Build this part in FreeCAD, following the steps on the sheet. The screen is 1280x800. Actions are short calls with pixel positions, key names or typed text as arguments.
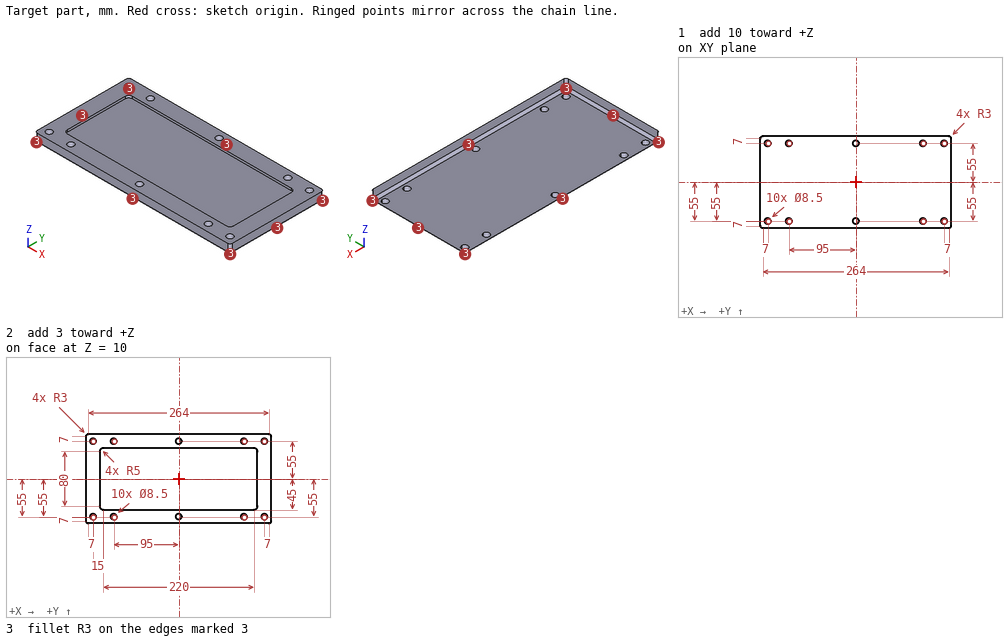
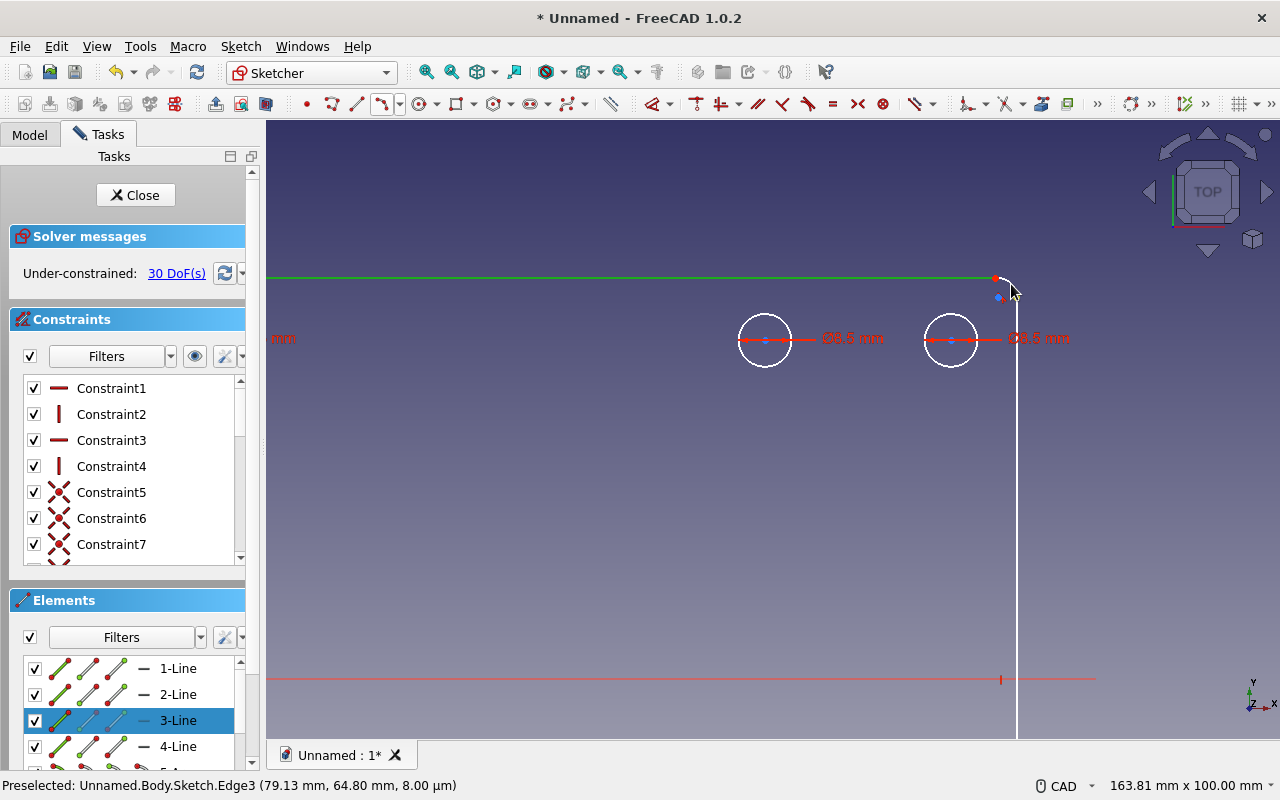
click(1010, 283)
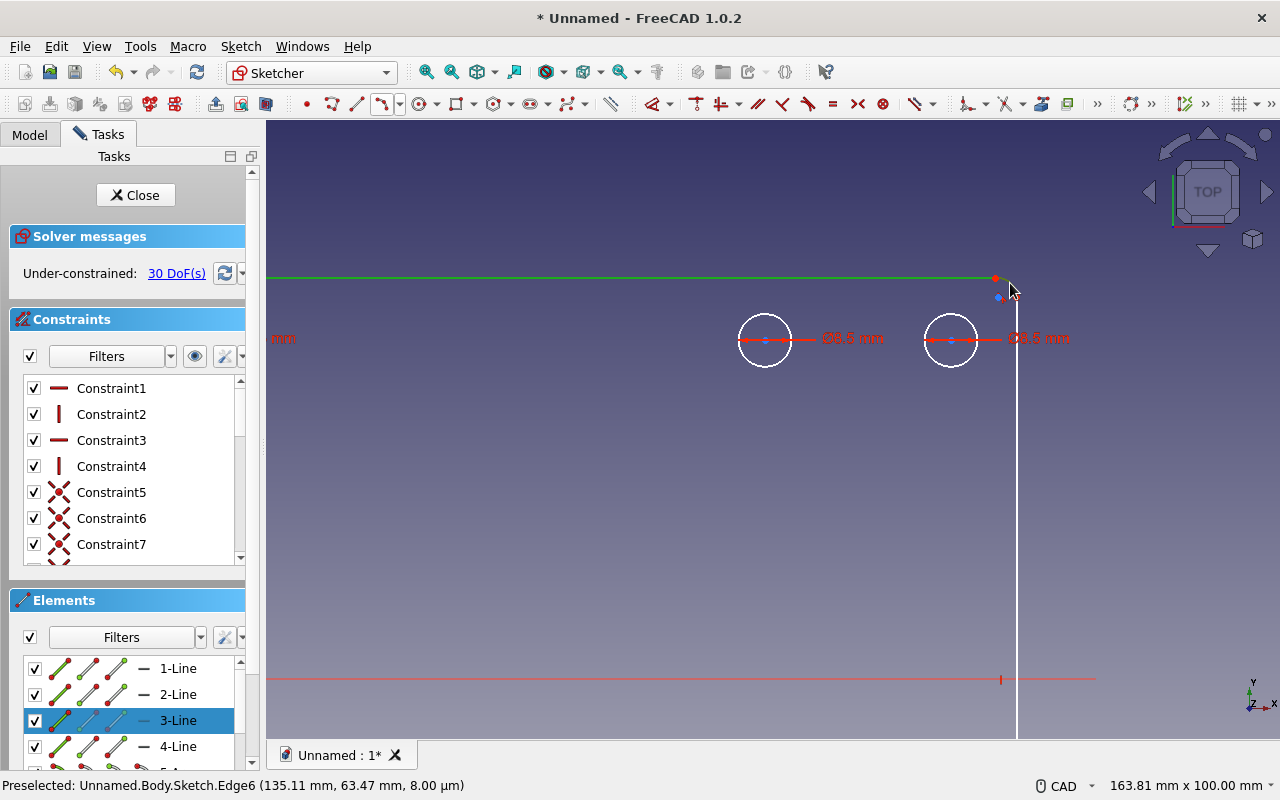
click(808, 104)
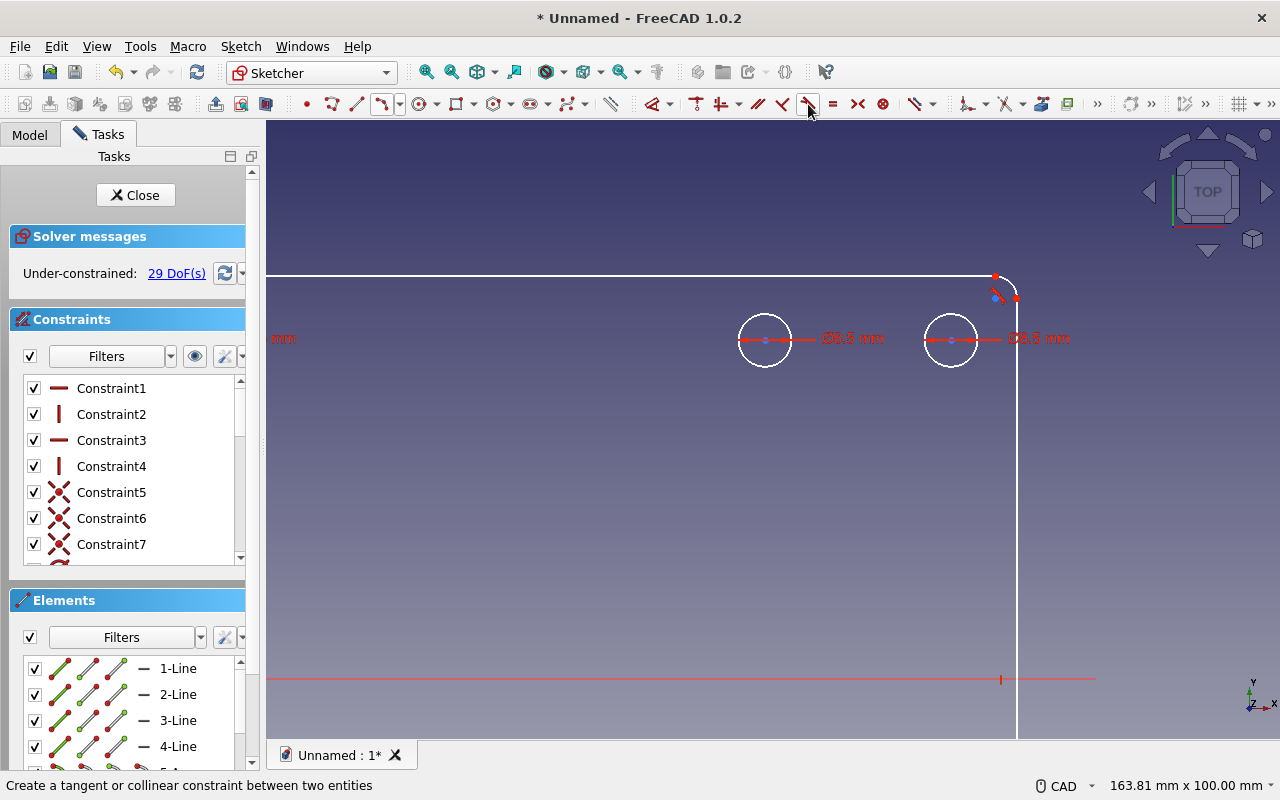
click(504, 276)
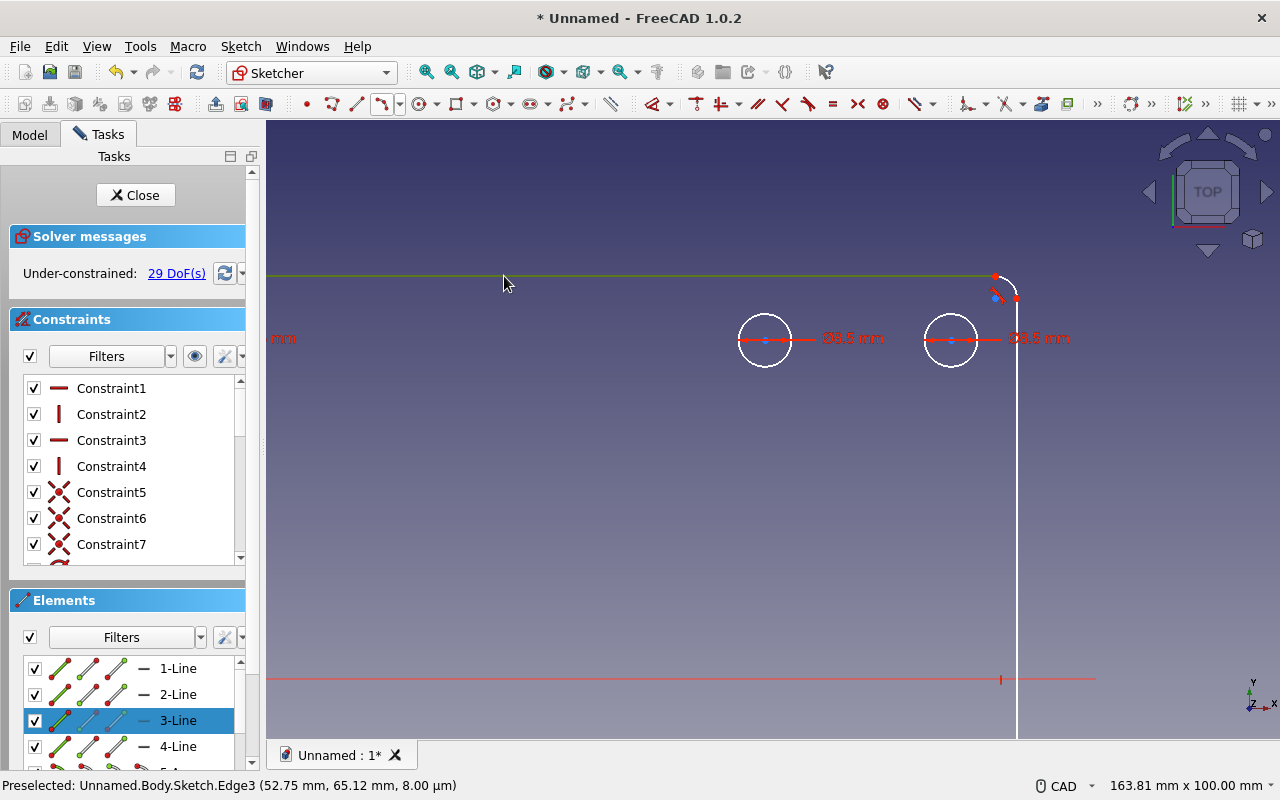
scroll(1011, 284, down, 5)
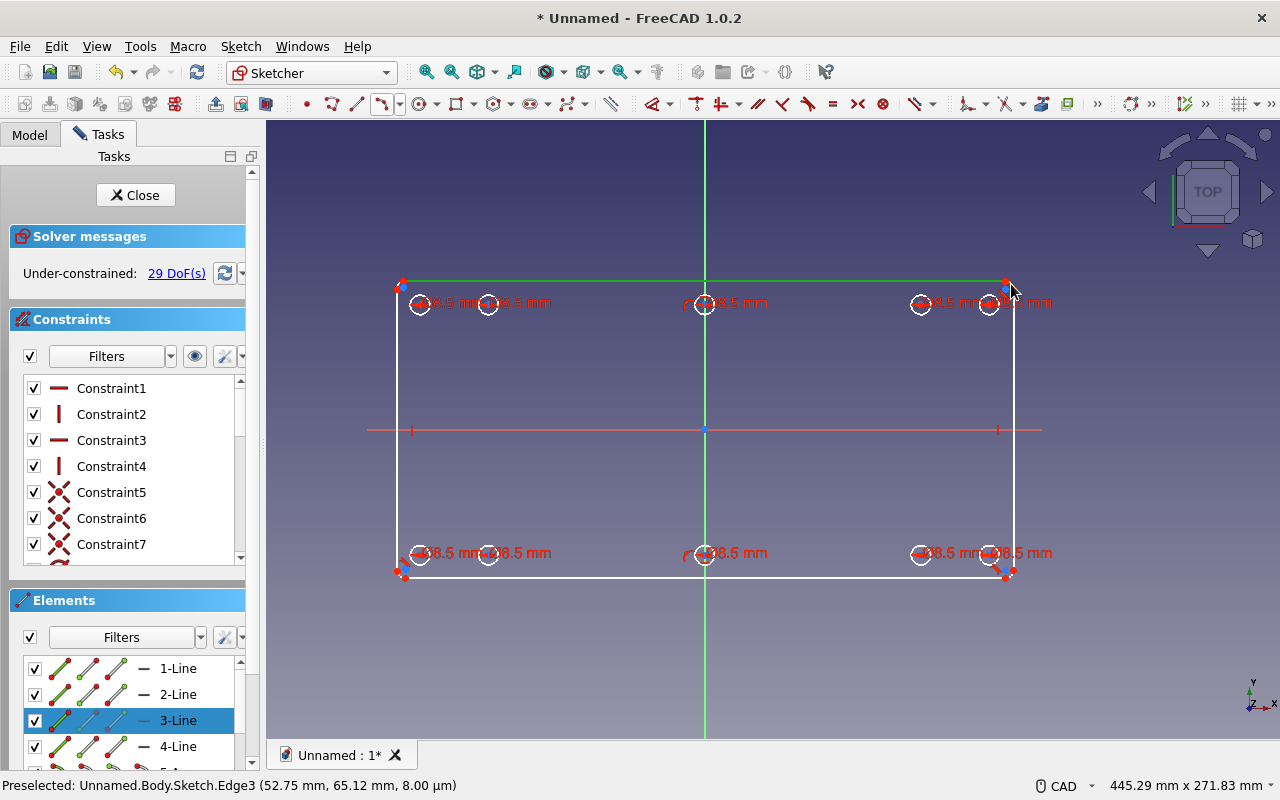
scroll(400, 282, up, 7)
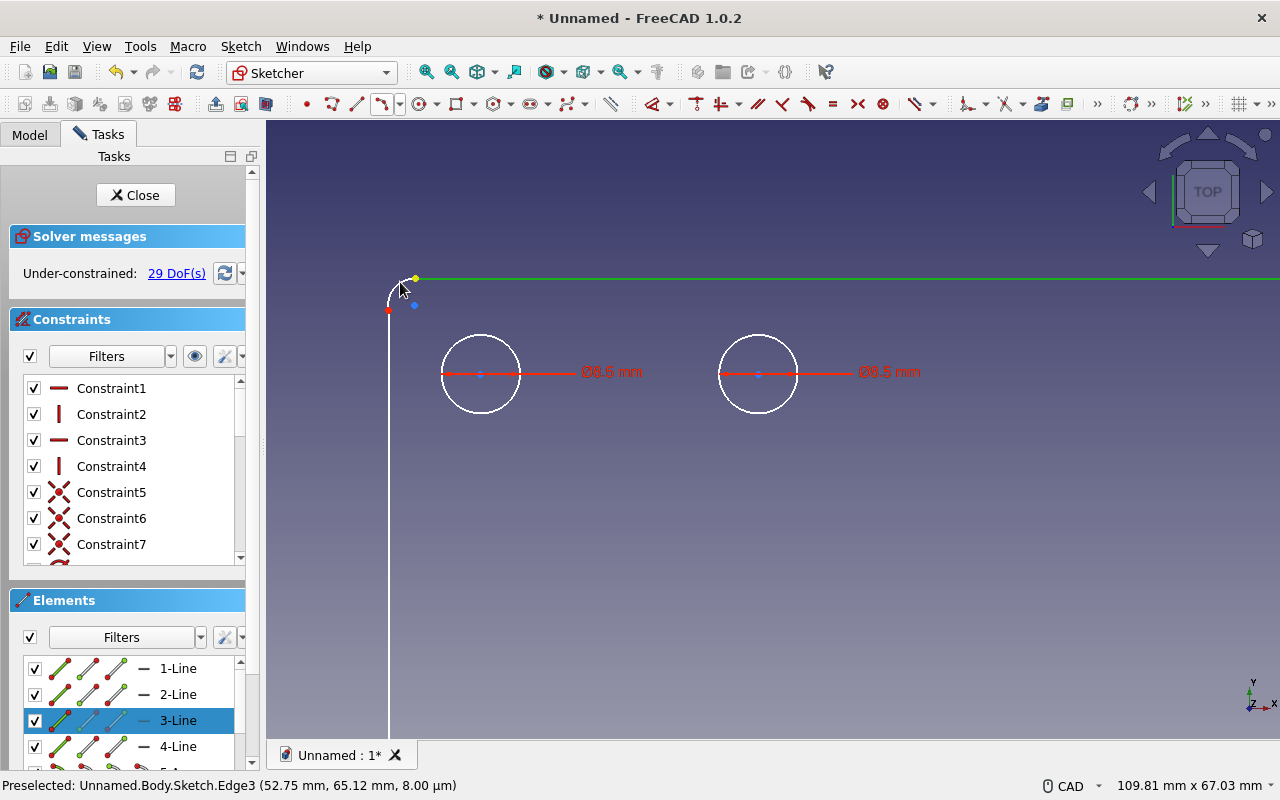
click(402, 282)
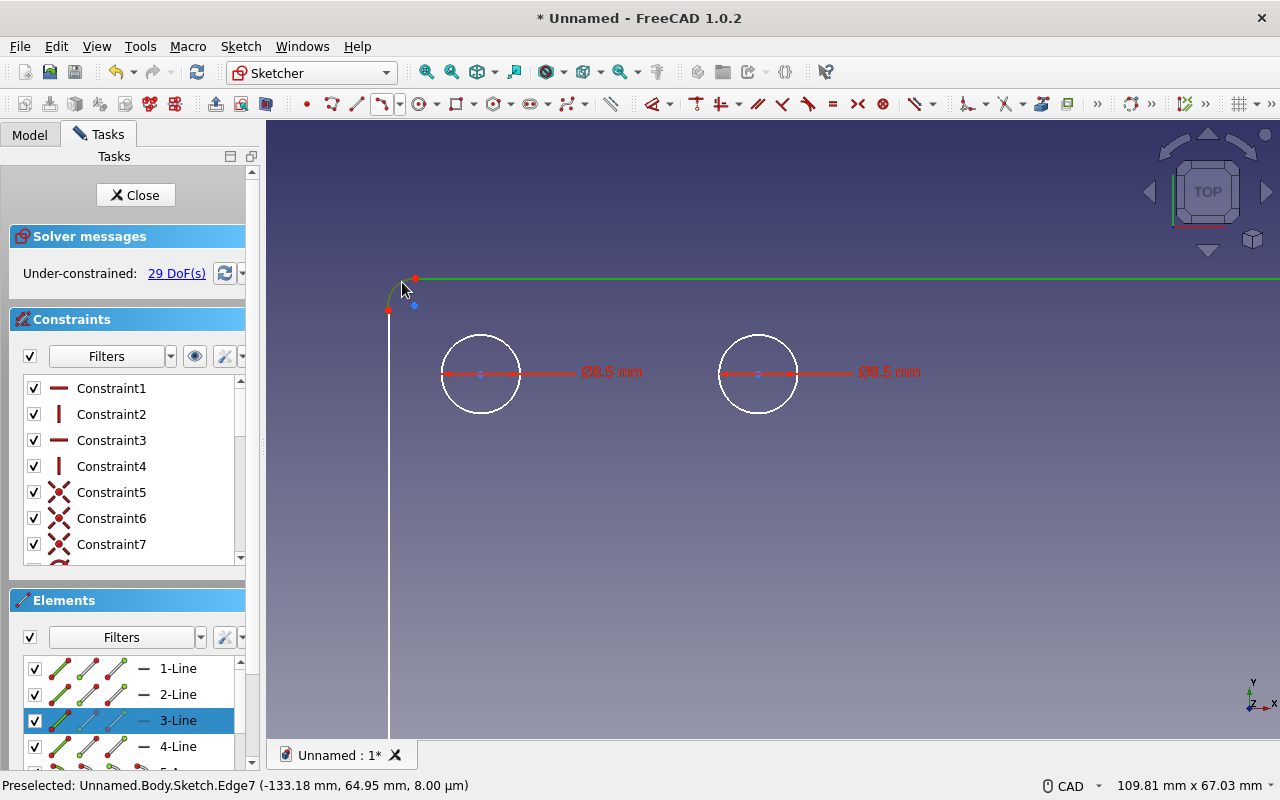
click(808, 104)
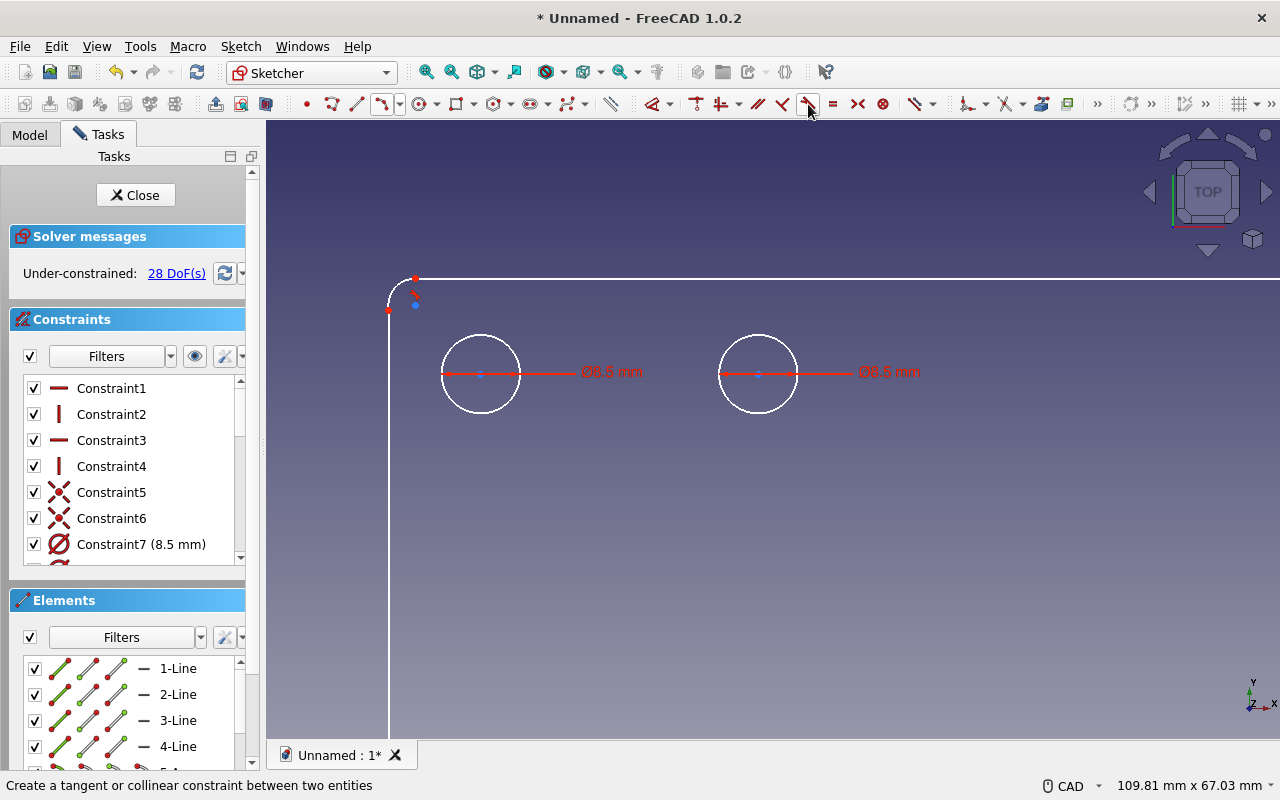
scroll(400, 282, down, 7)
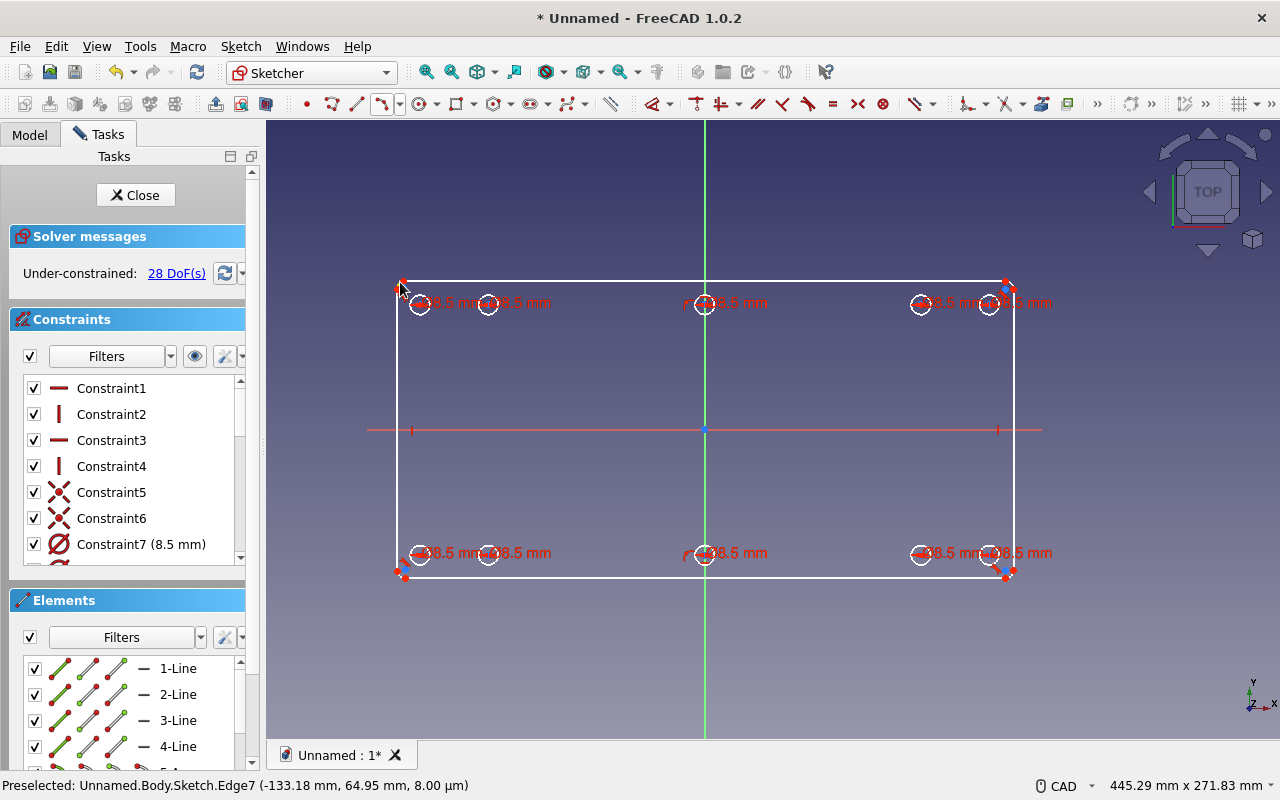
click(397, 374)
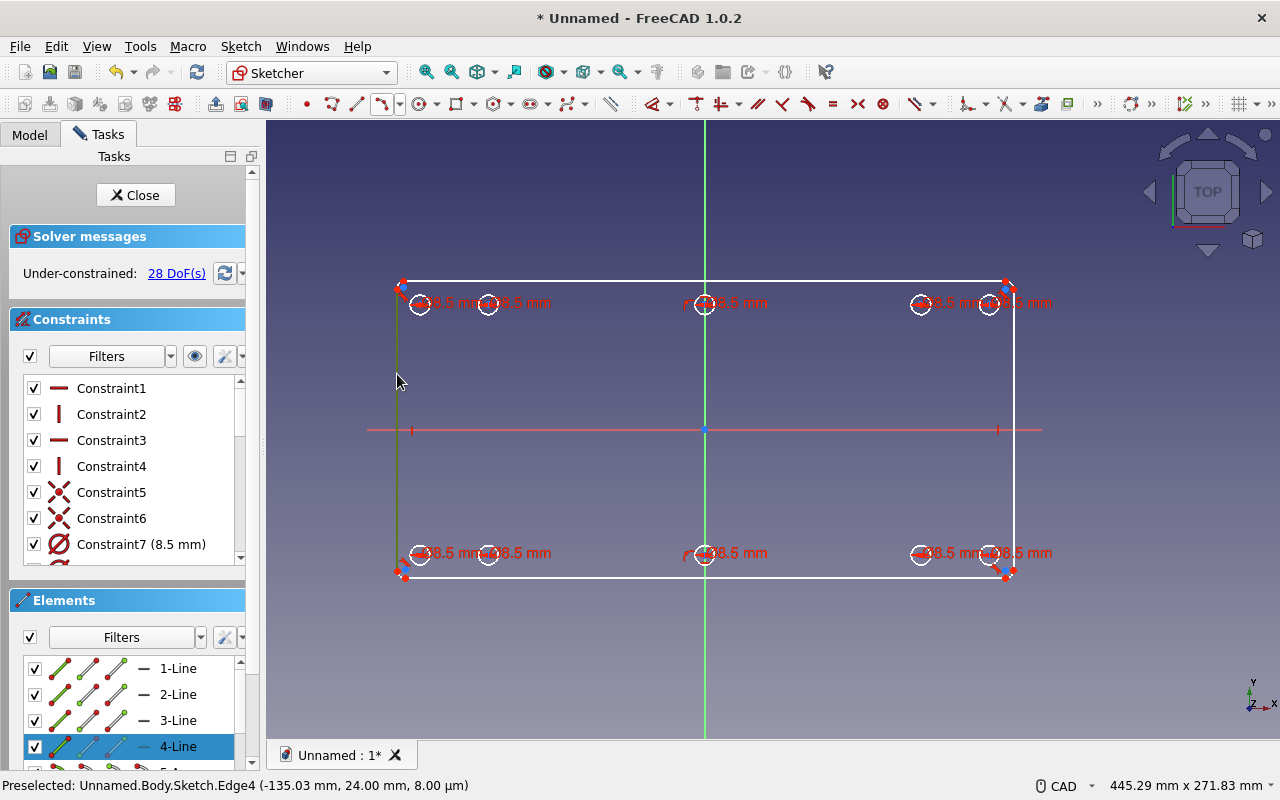
scroll(399, 284, up, 5)